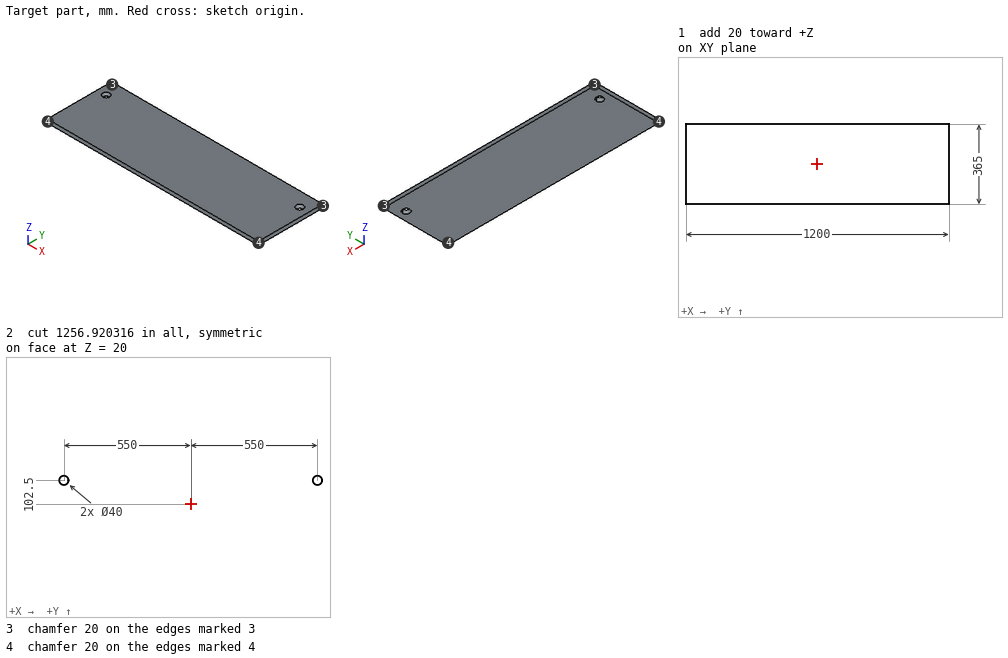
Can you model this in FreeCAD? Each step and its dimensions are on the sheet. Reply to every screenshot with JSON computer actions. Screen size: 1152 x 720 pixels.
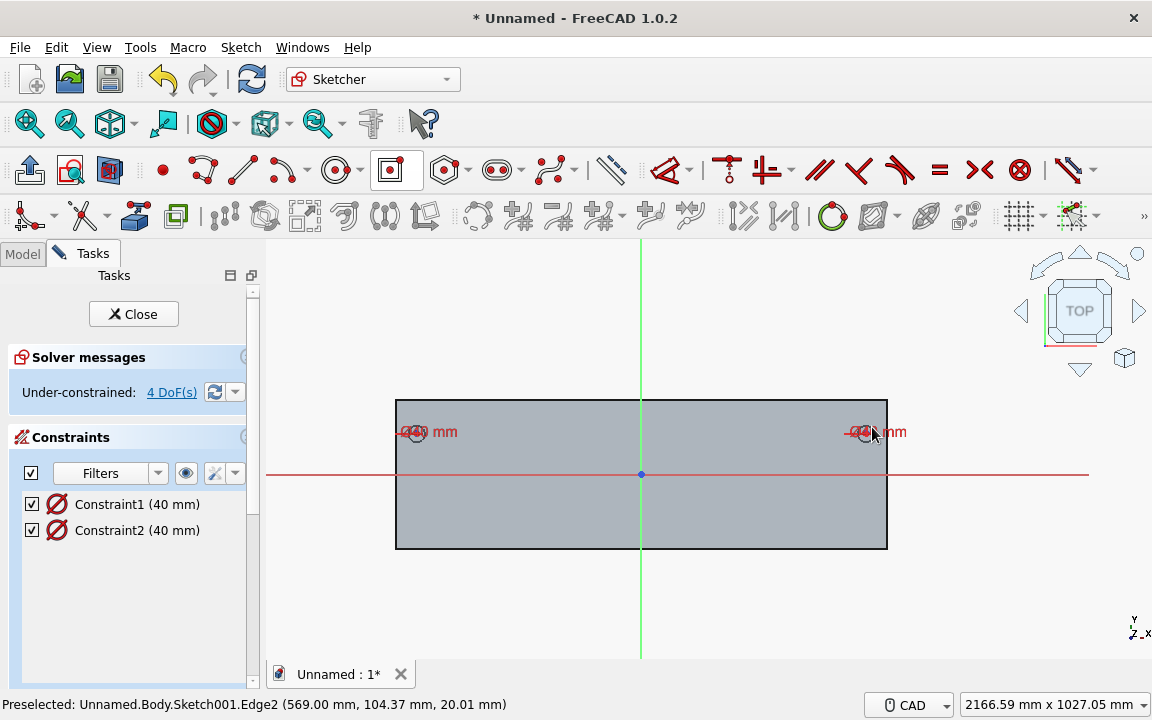
{"action": "left_click", "coordinate": [417, 434]}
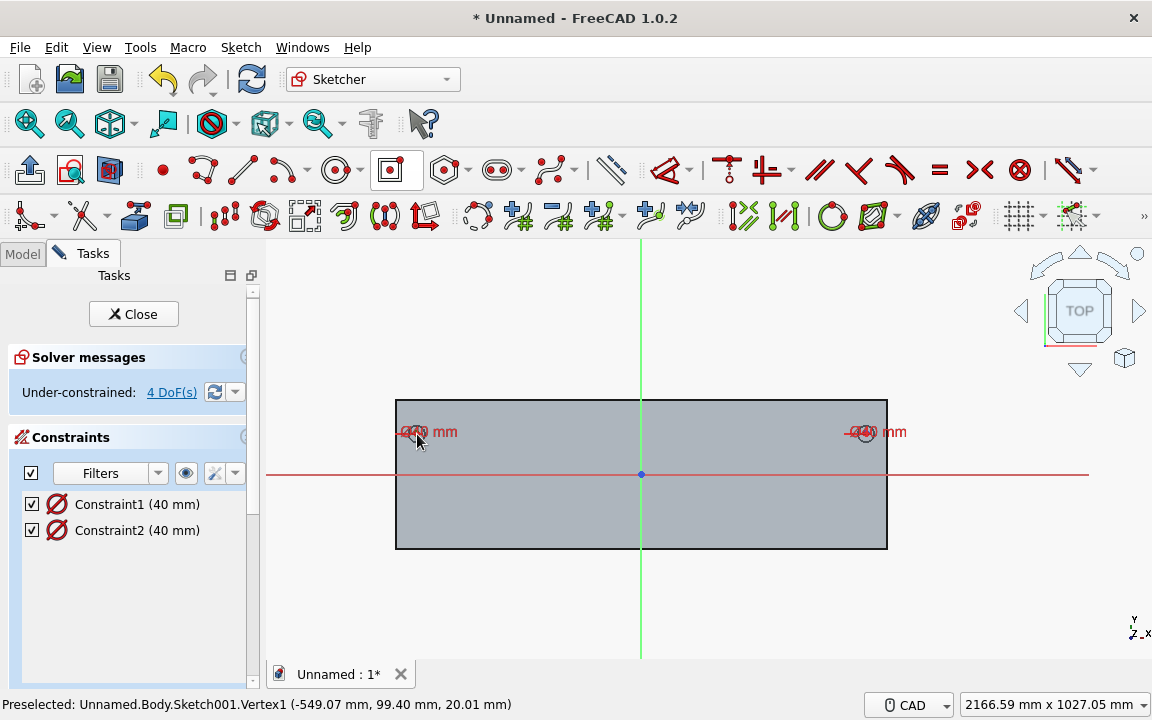
{"action": "left_click", "coordinate": [866, 434]}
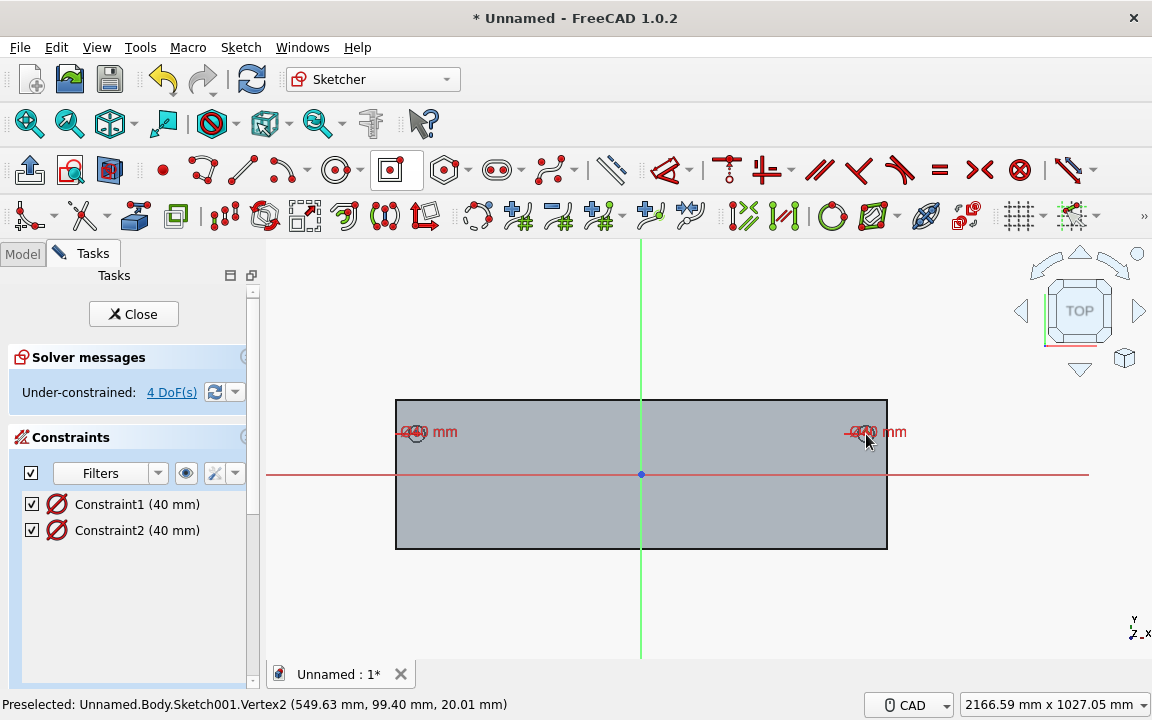
{"action": "key", "text": "h"}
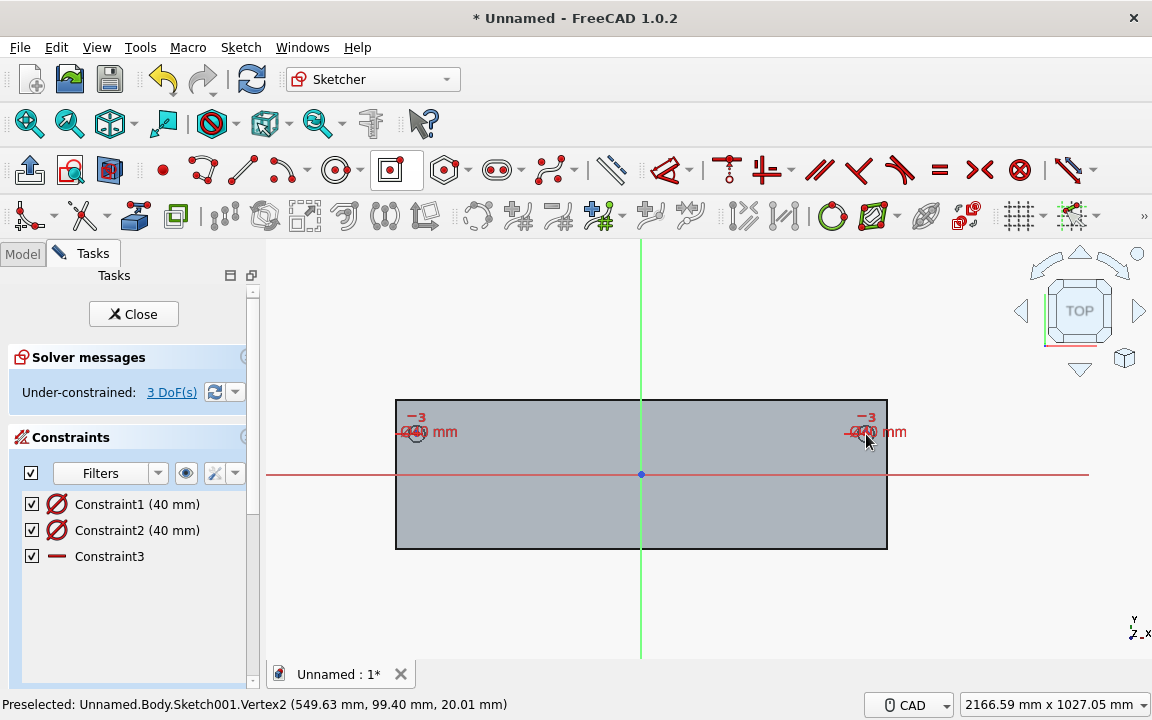
{"action": "left_click", "coordinate": [417, 434]}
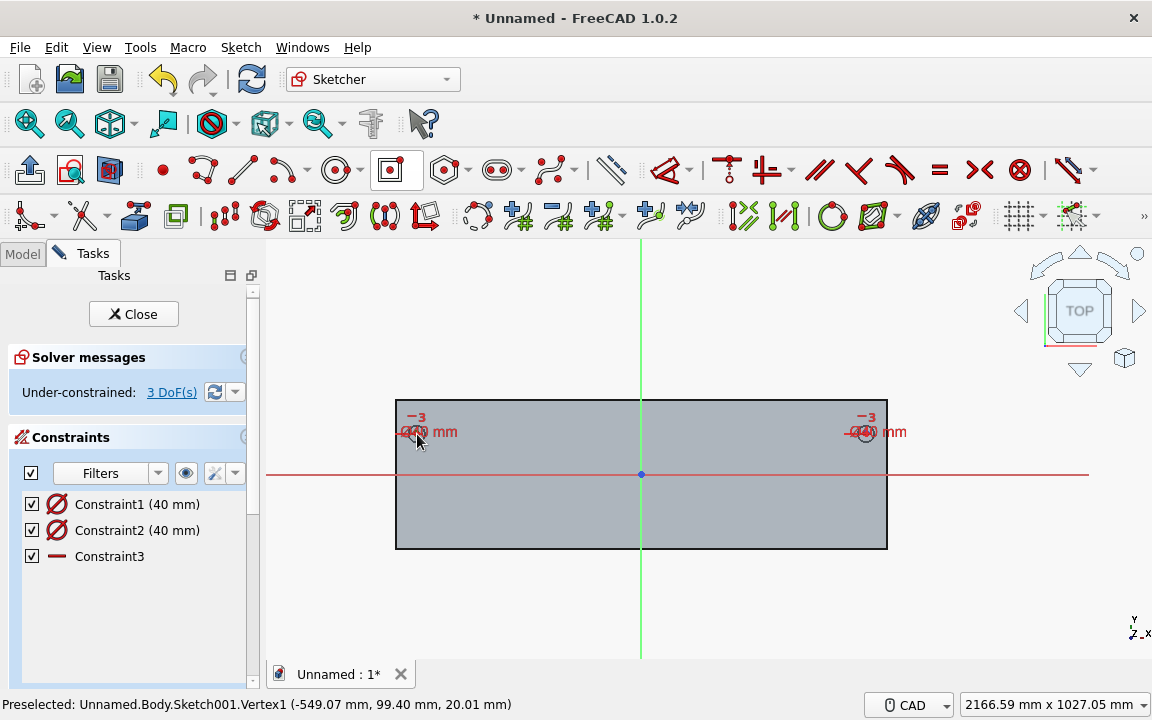
{"action": "key", "text": "l"}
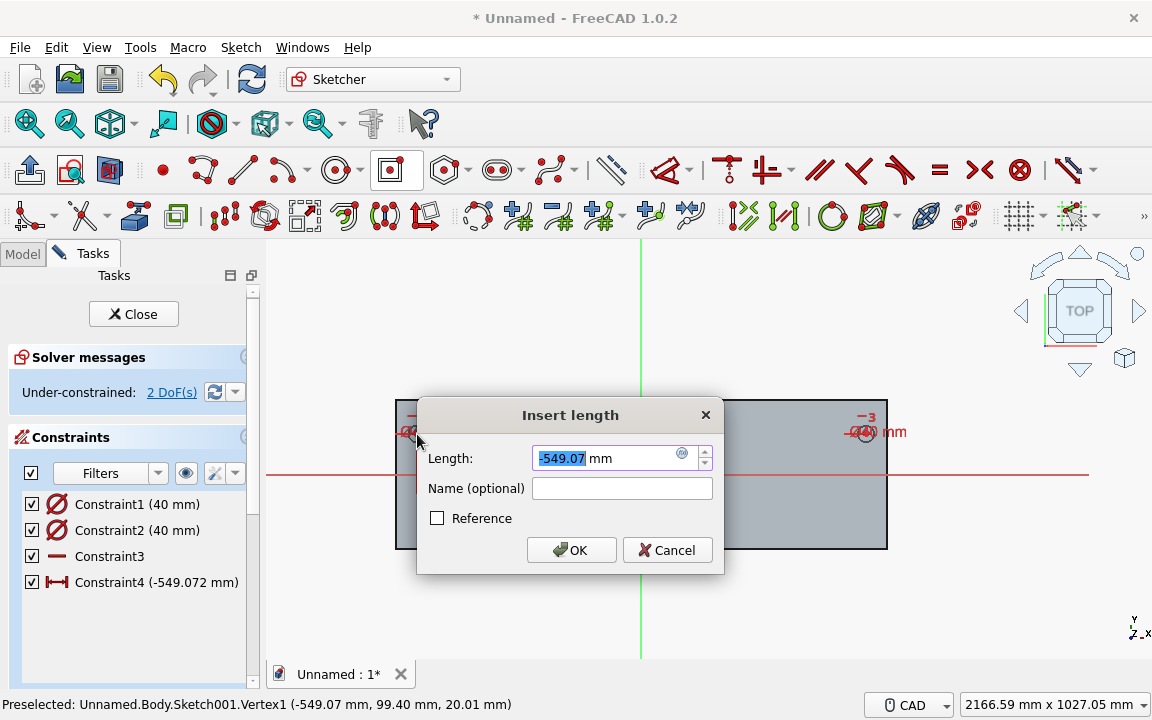
{"action": "type", "text": "-550"}
{"action": "key", "text": "Return"}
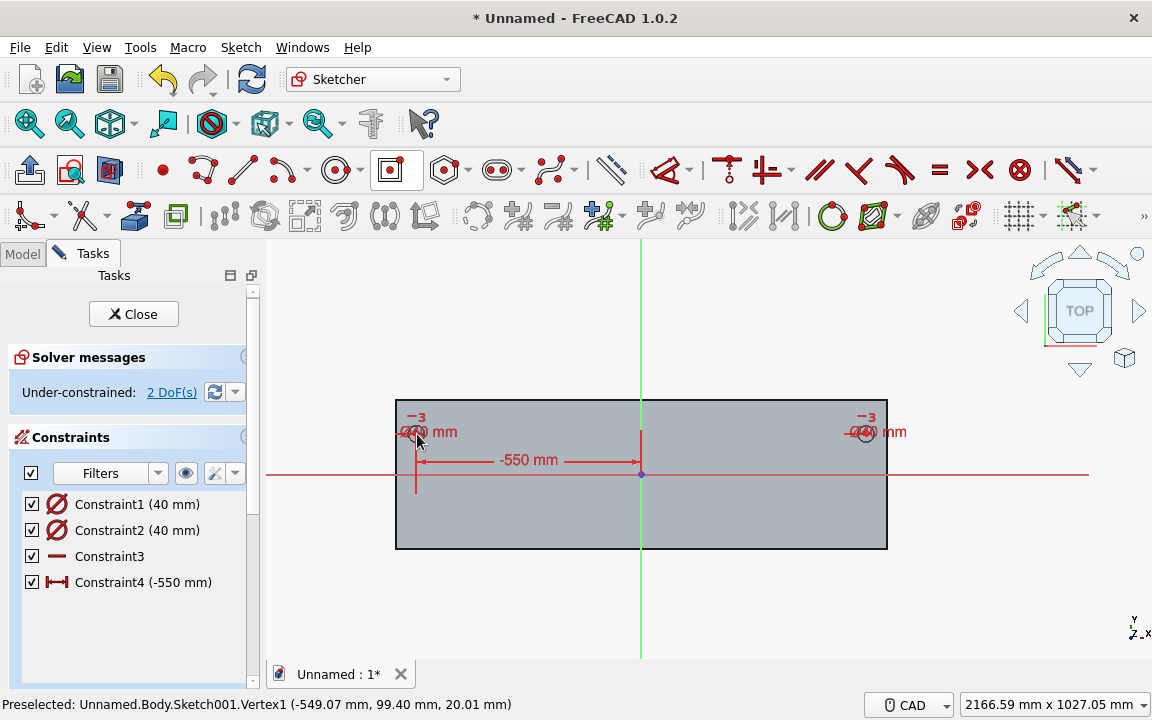
{"action": "left_click", "coordinate": [866, 434]}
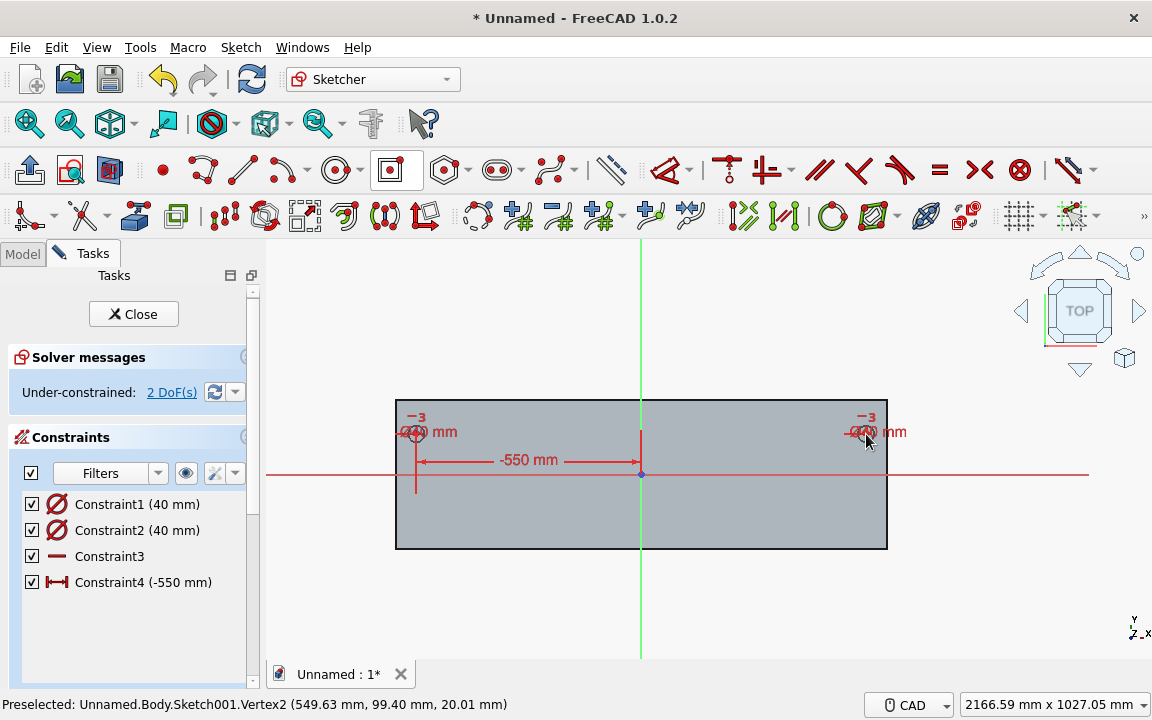
{"action": "key", "text": "l"}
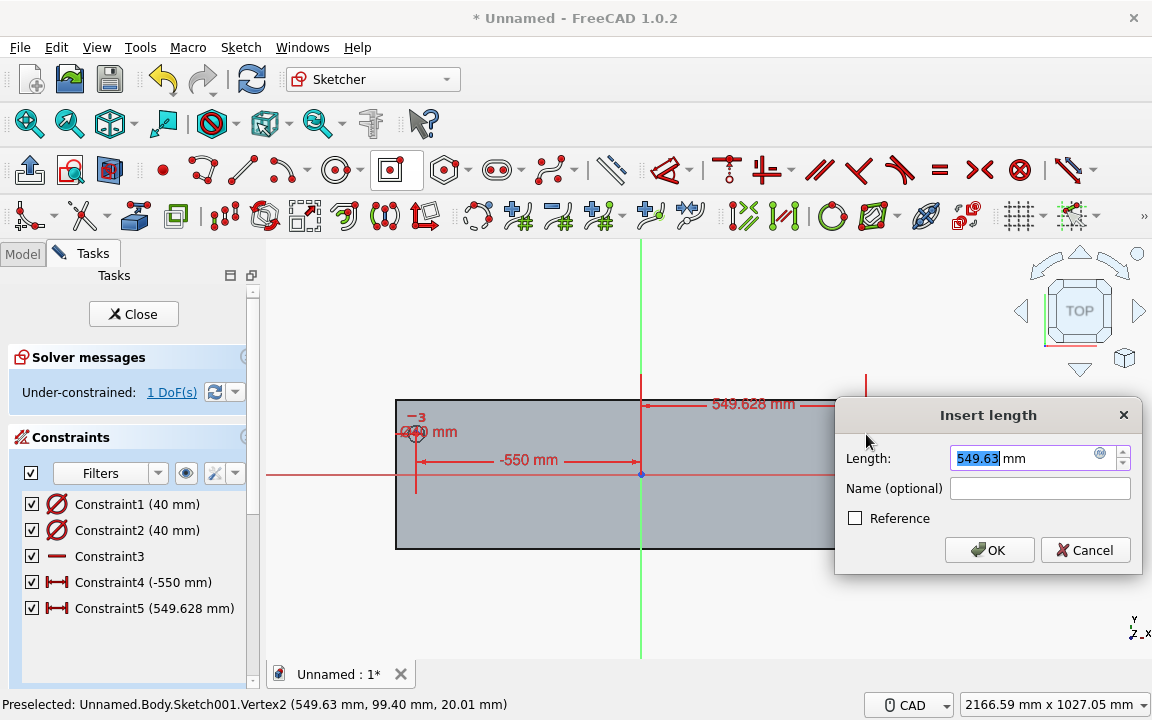
{"action": "type", "text": "550"}
{"action": "key", "text": "Return"}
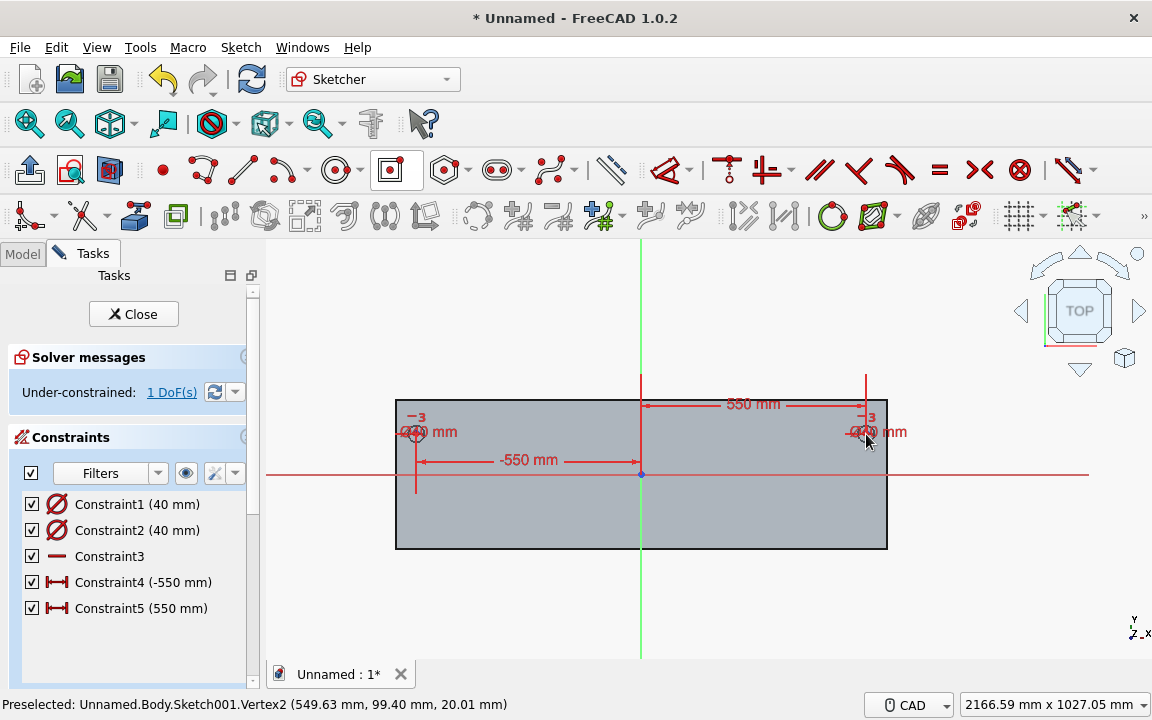
{"action": "left_click", "coordinate": [416, 434]}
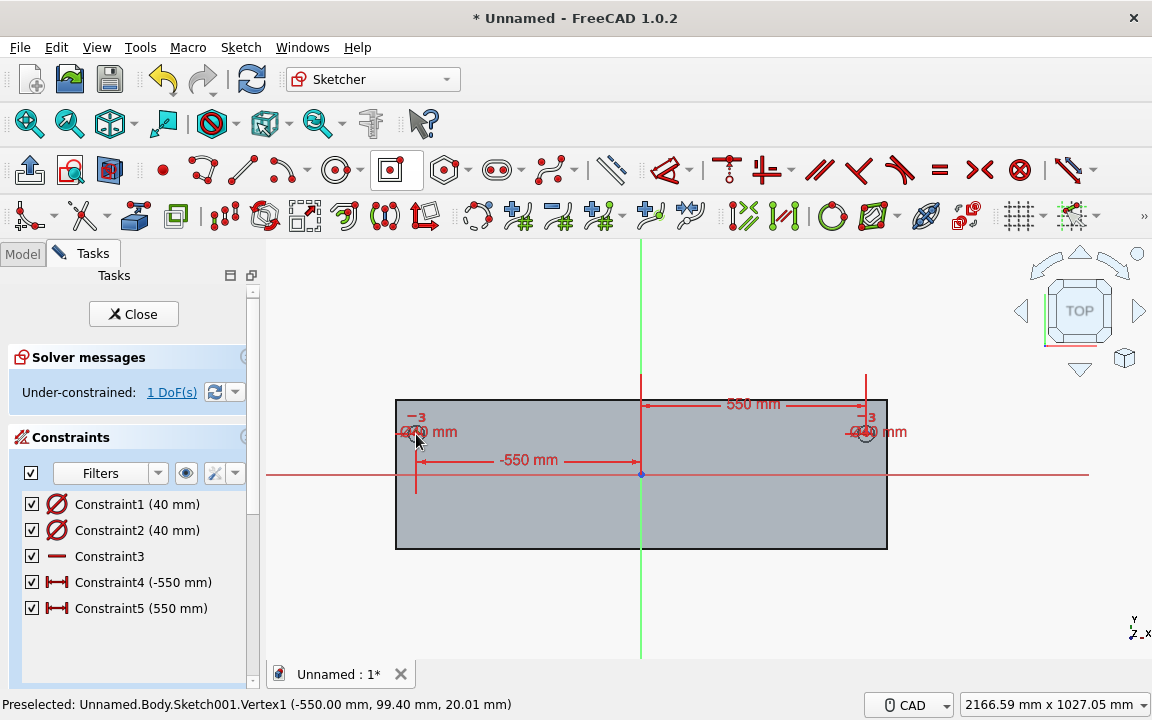
{"action": "key", "text": "i"}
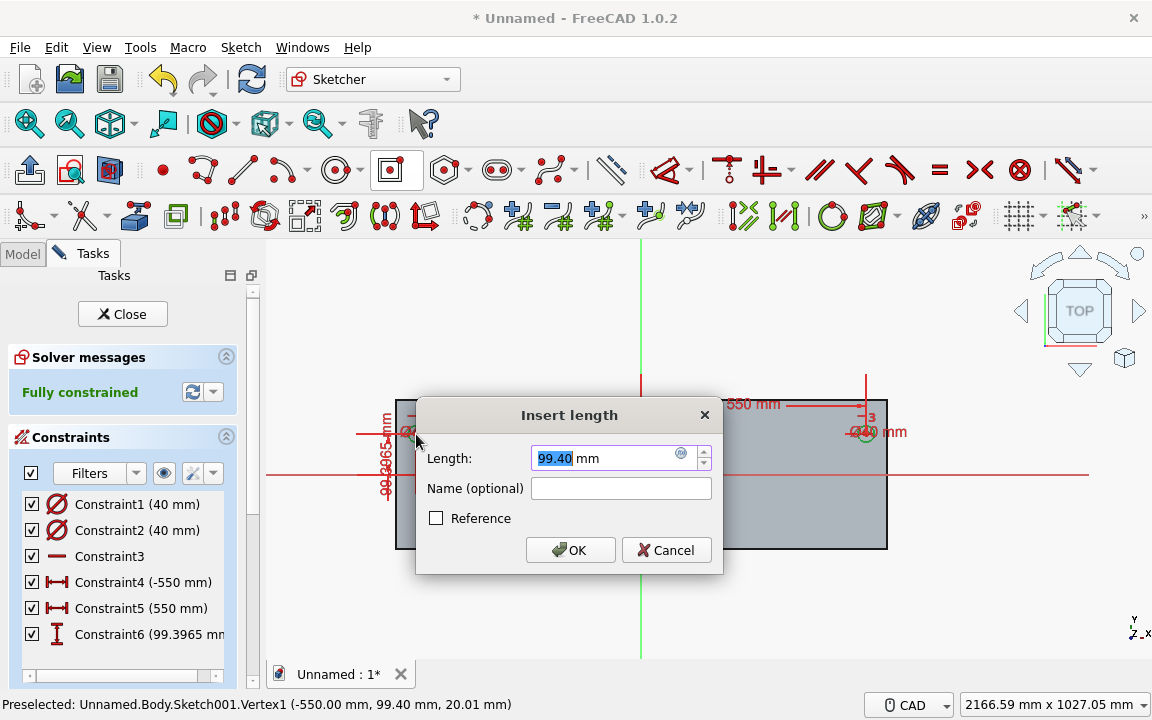
{"action": "type", "text": "102.5"}
{"action": "key", "text": "Return"}